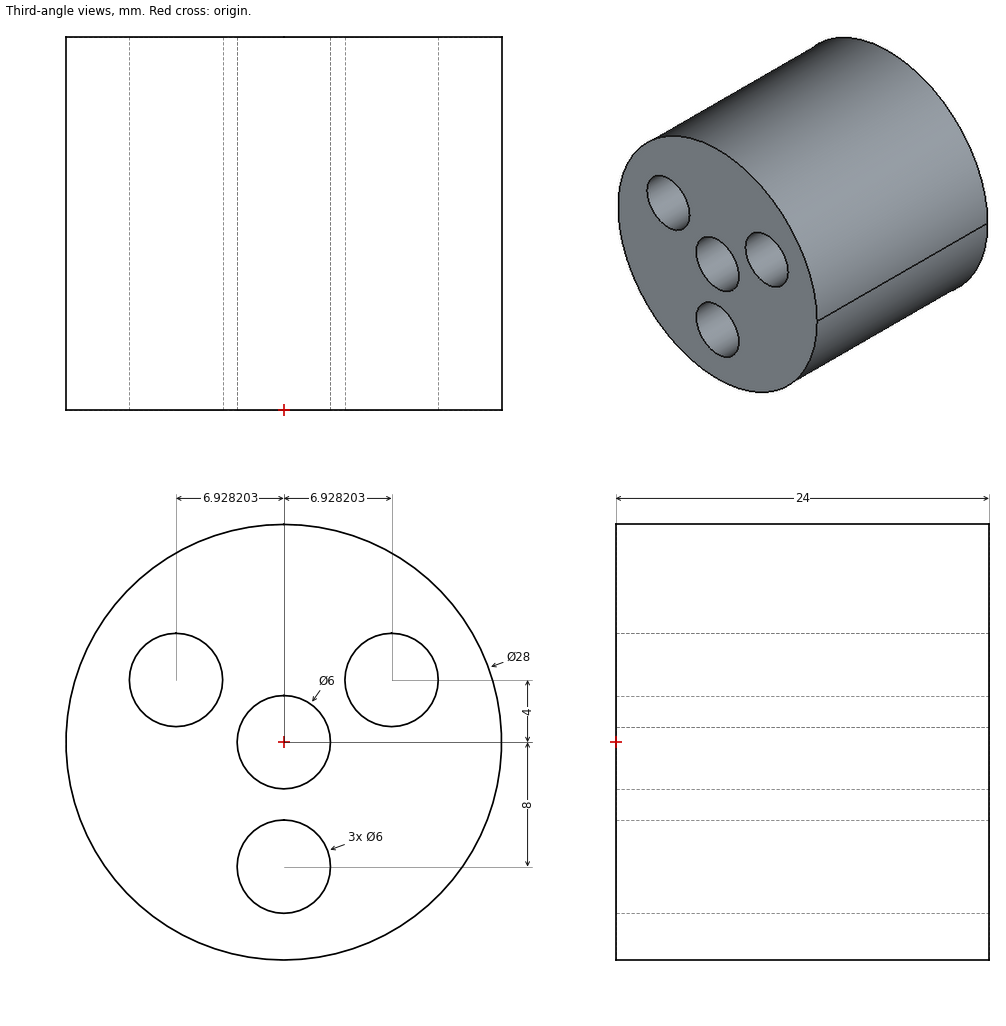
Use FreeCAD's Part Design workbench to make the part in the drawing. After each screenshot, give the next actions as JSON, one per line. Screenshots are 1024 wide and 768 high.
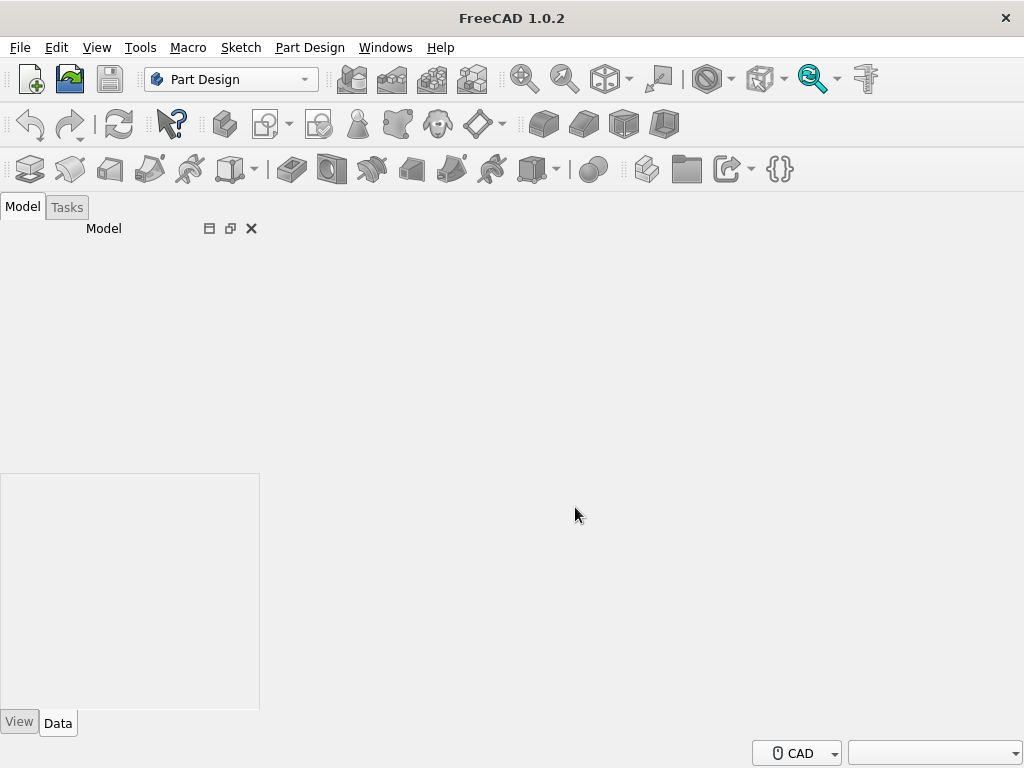
{"action": "left_click", "coordinate": [30, 80]}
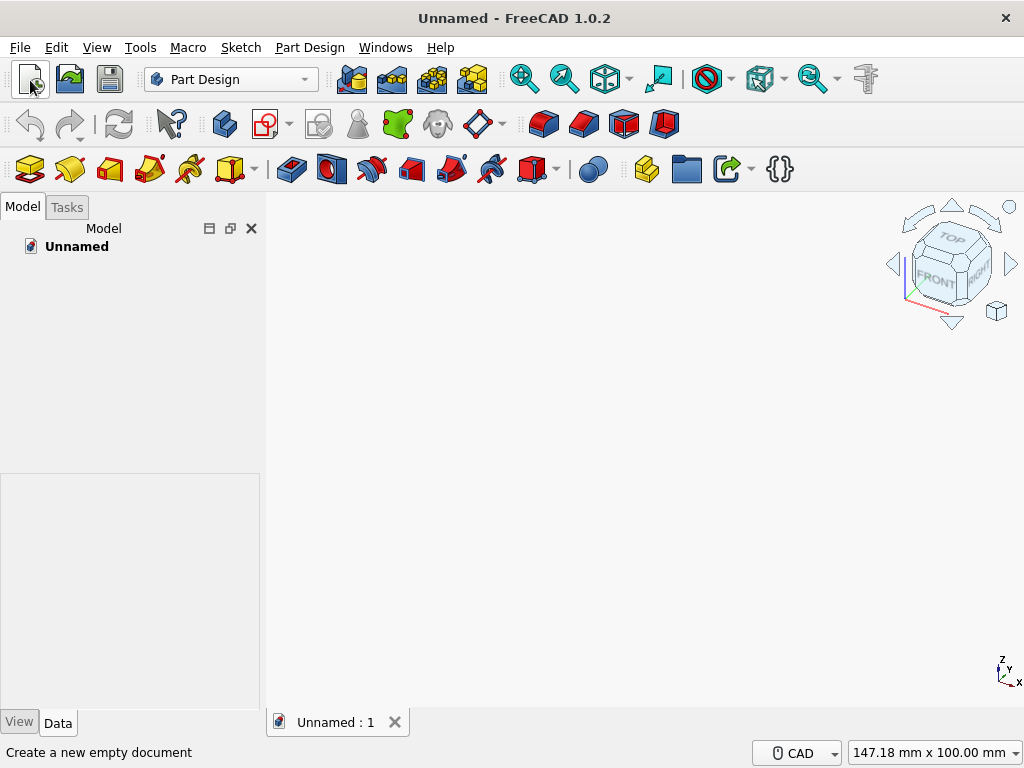
{"action": "left_click", "coordinate": [266, 124]}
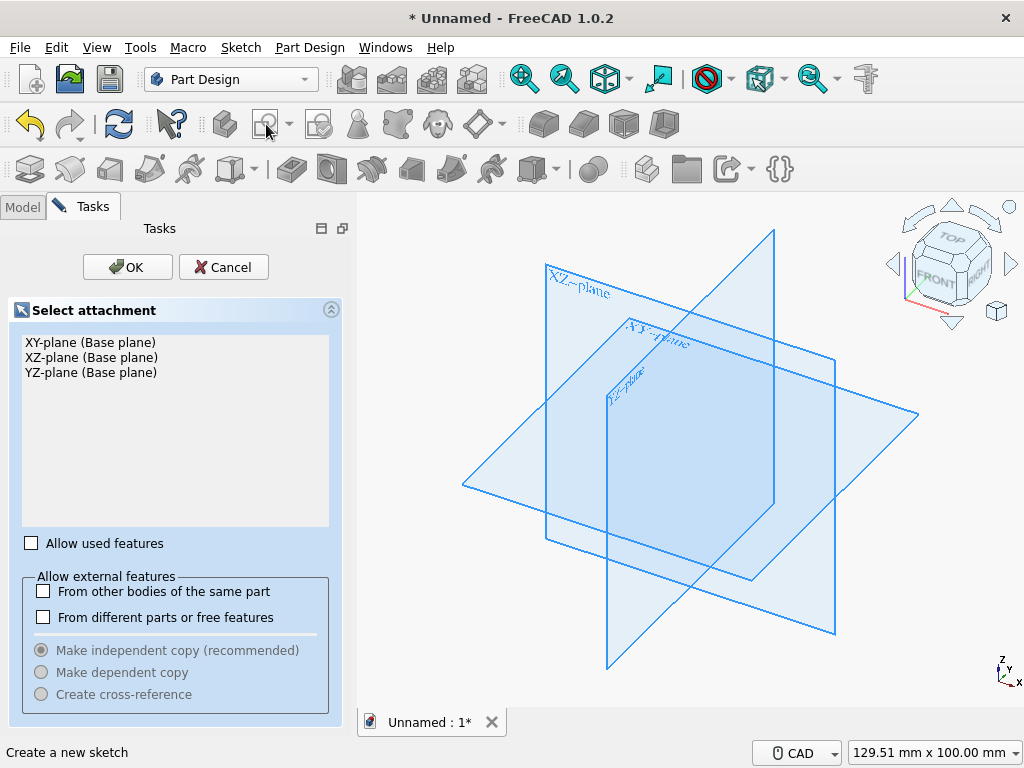
{"action": "left_click", "coordinate": [82, 358]}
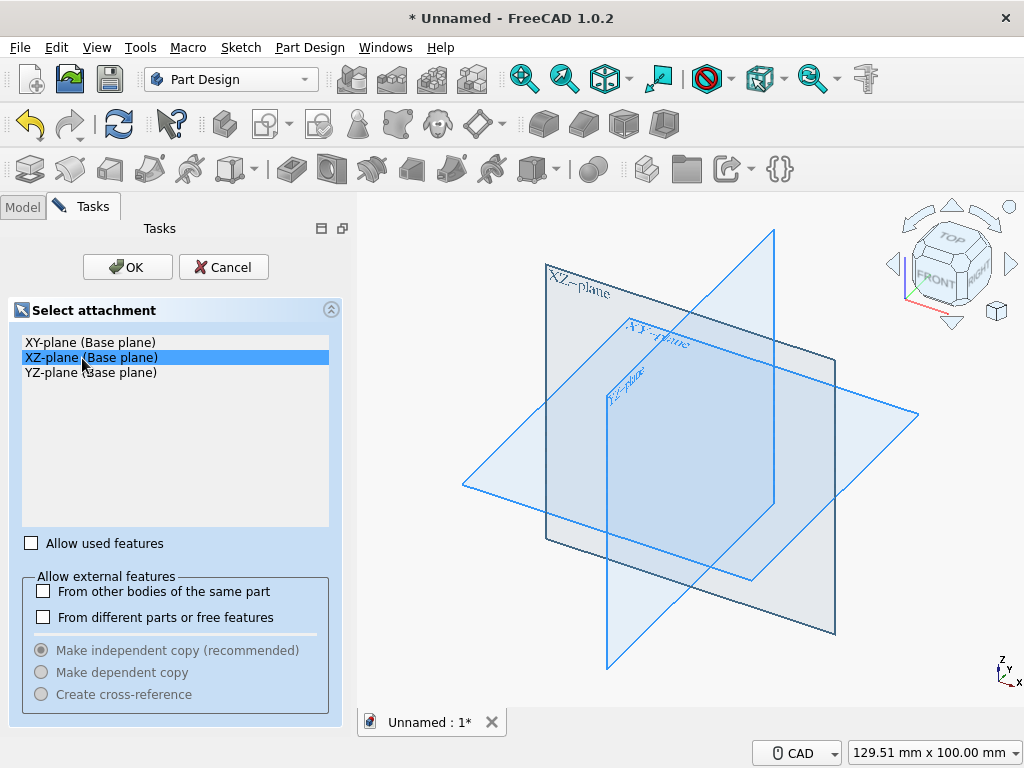
{"action": "left_click", "coordinate": [128, 267]}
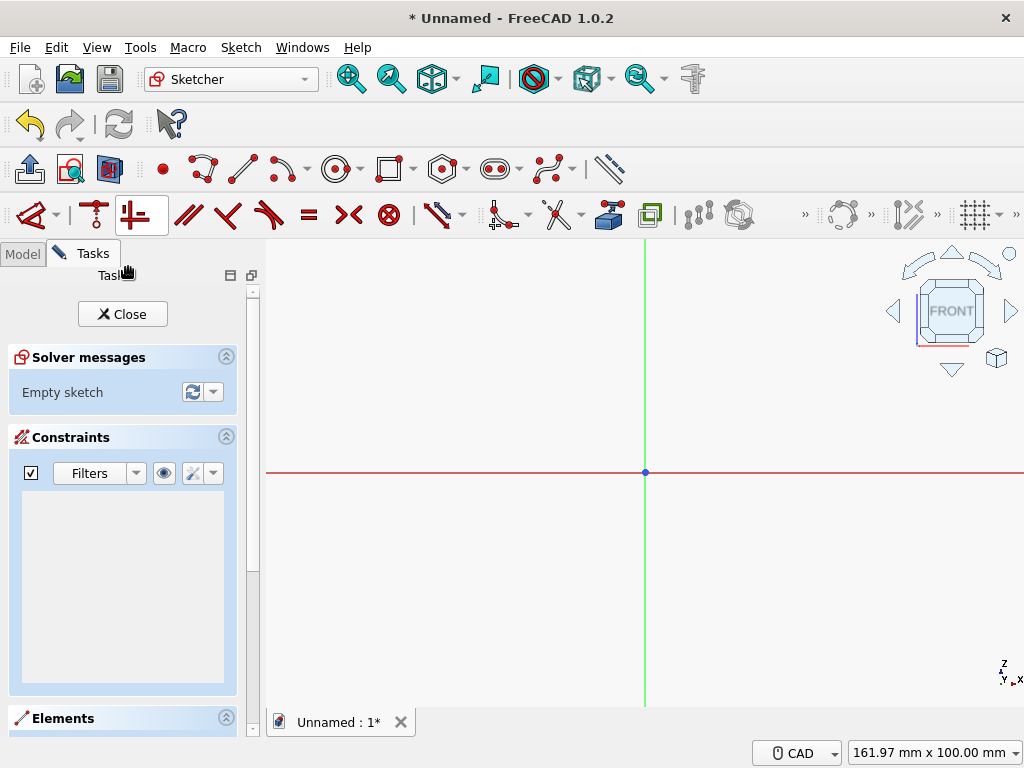
{"action": "scroll", "coordinate": [701, 473], "scroll_direction": "up", "scroll_amount": 4}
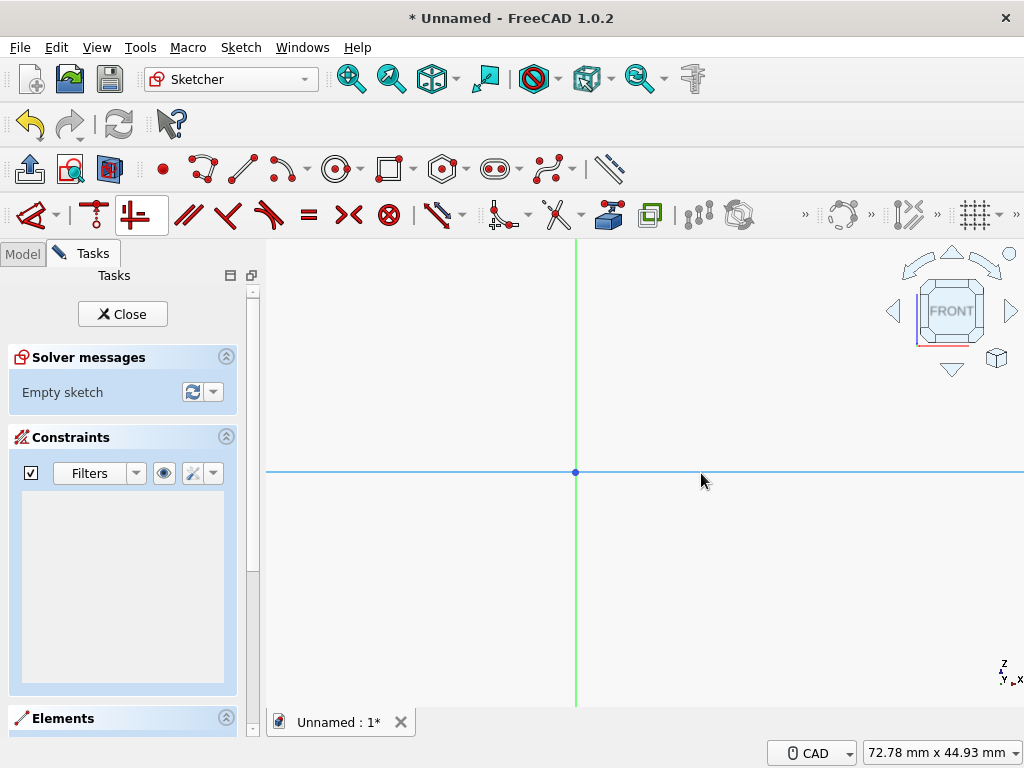
{"action": "left_click", "coordinate": [336, 170]}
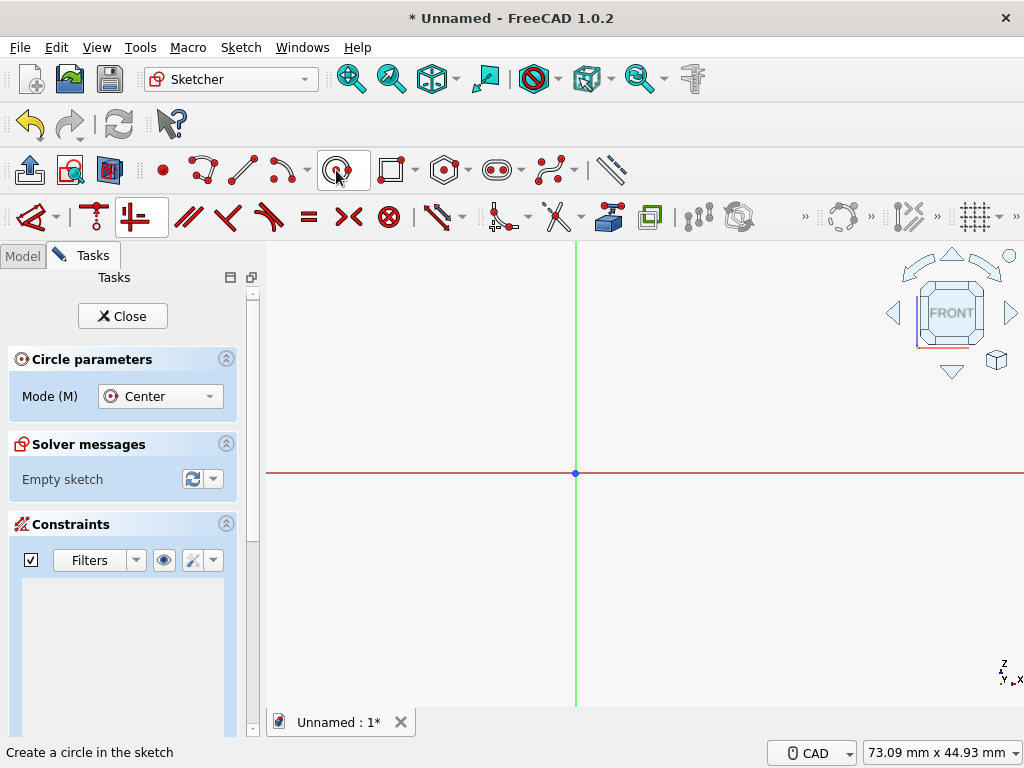
{"action": "left_click", "coordinate": [576, 473]}
{"action": "mouse_move", "coordinate": [679, 371]}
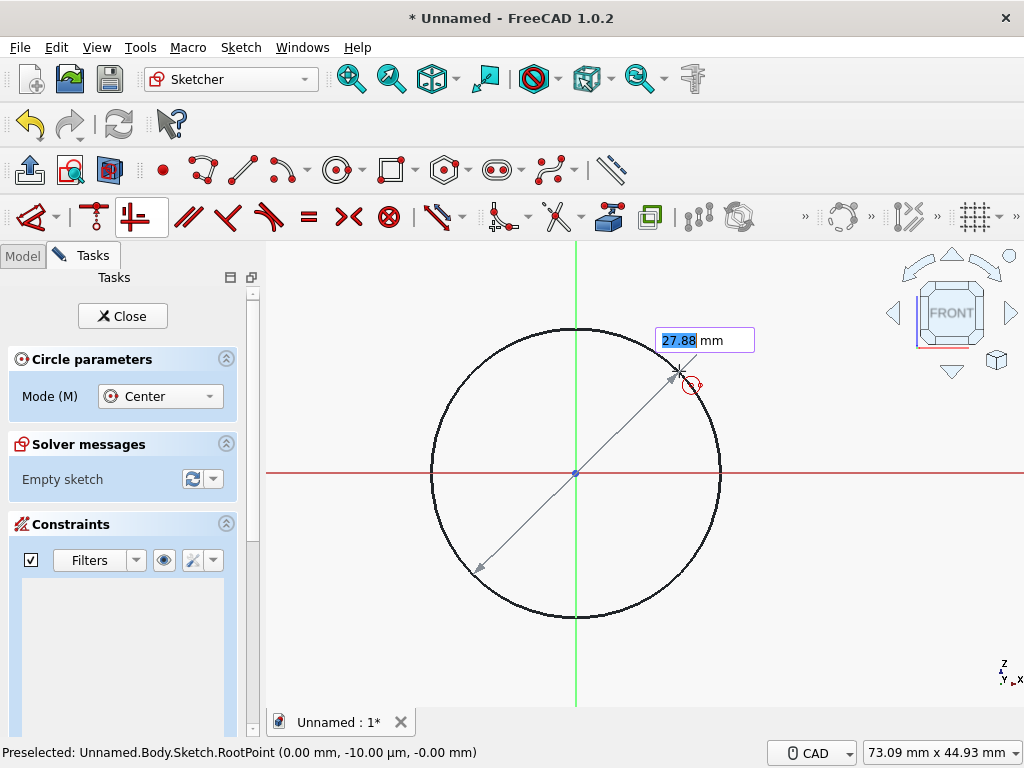
{"action": "type", "text": "28"}
{"action": "key", "text": "Return"}
{"action": "key", "text": "Escape"}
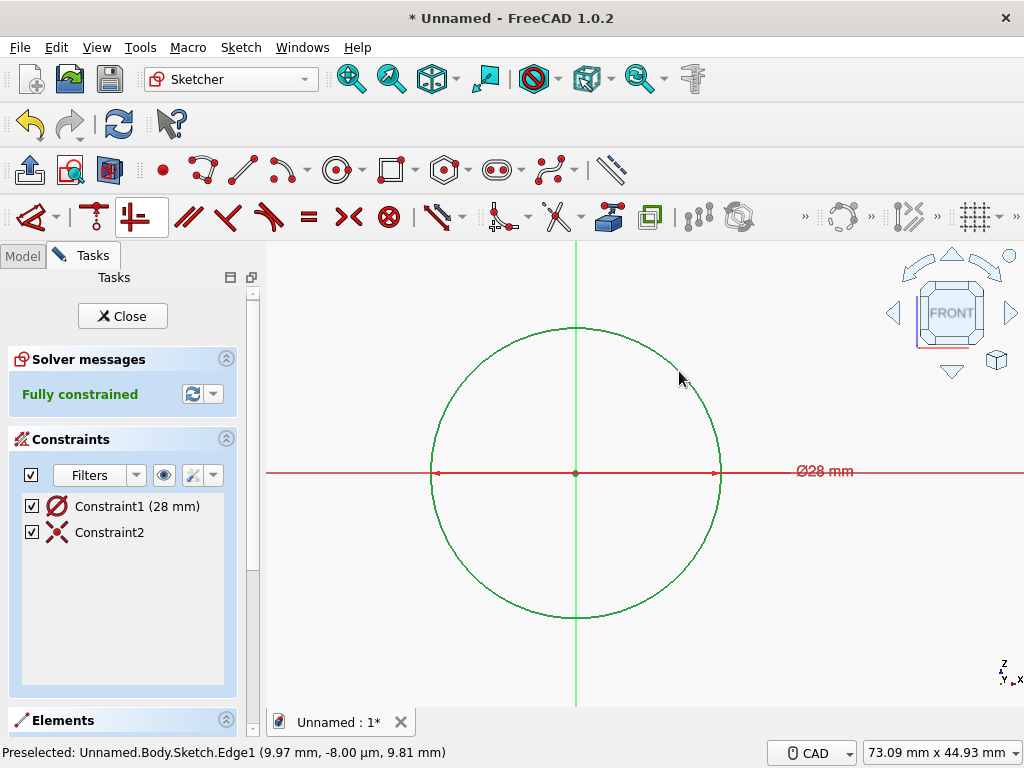
{"action": "left_click", "coordinate": [123, 316]}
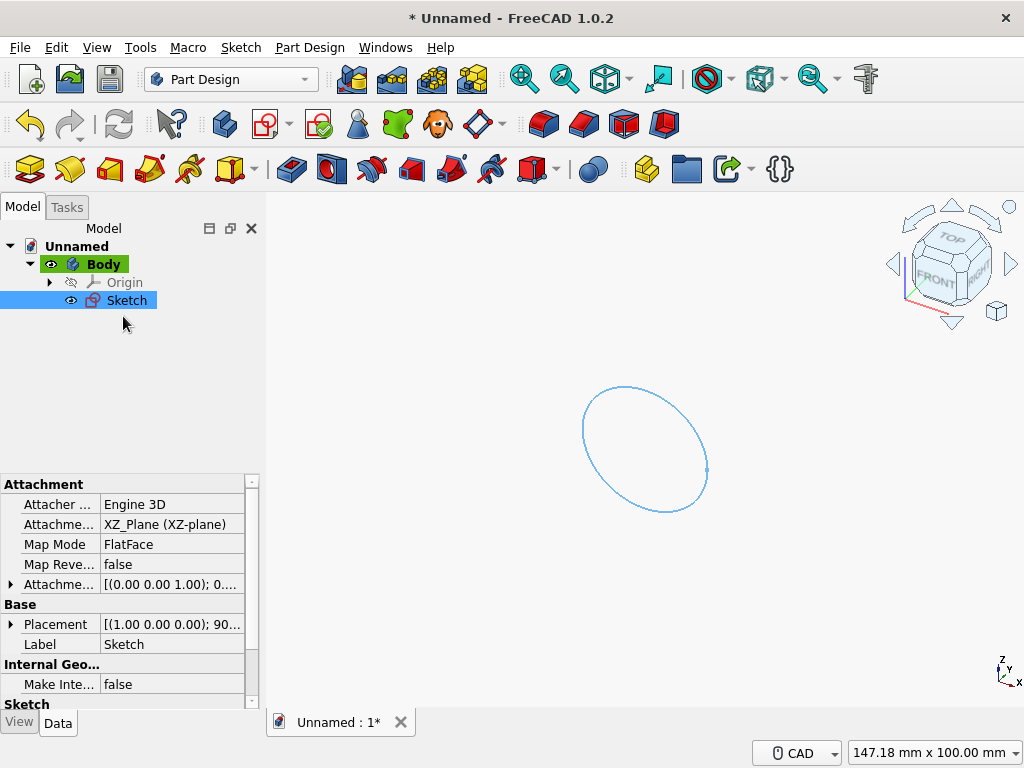
{"action": "left_click", "coordinate": [30, 170]}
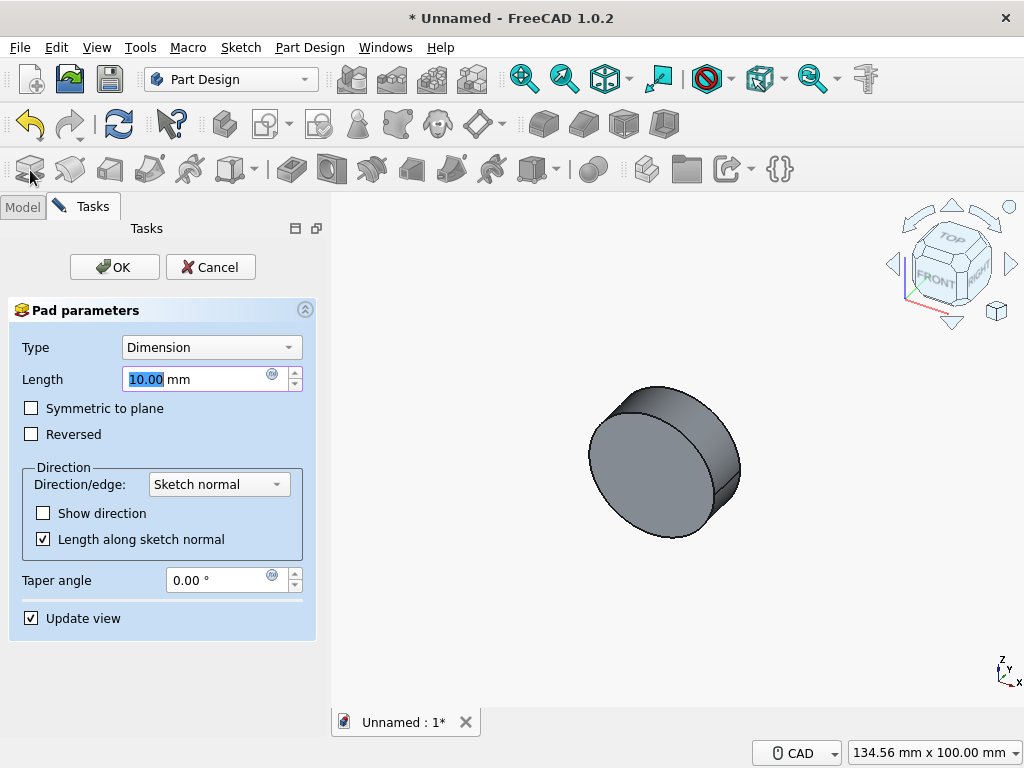
{"action": "type", "text": "24"}
{"action": "key", "text": "Tab"}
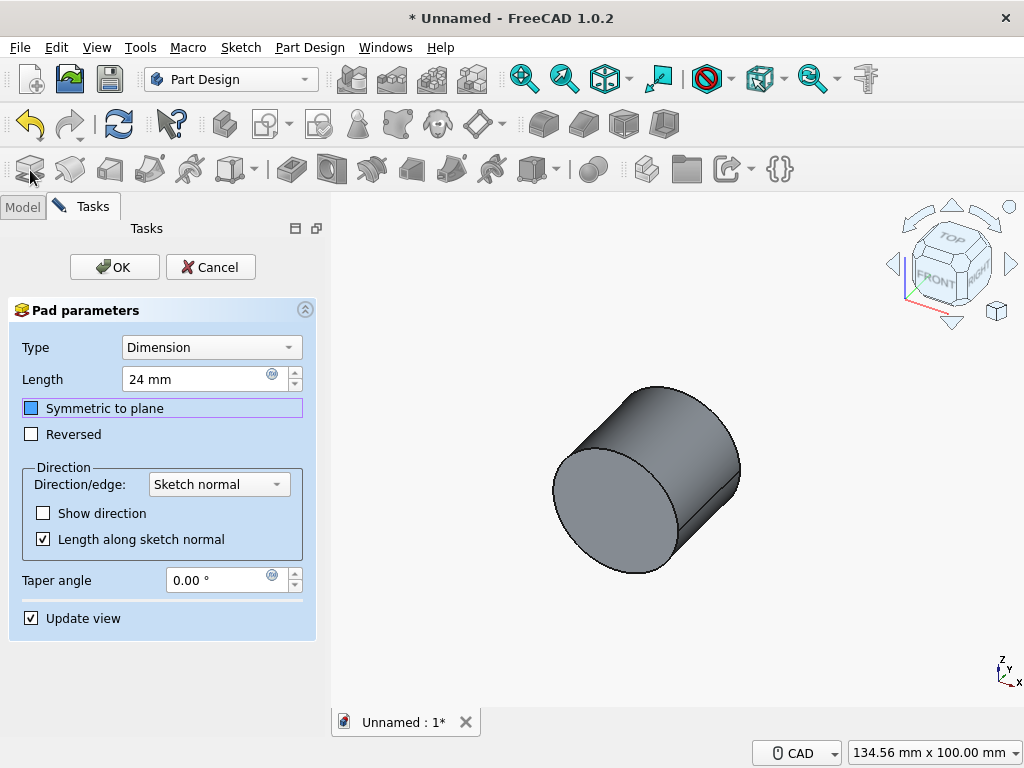
{"action": "left_click", "coordinate": [30, 434]}